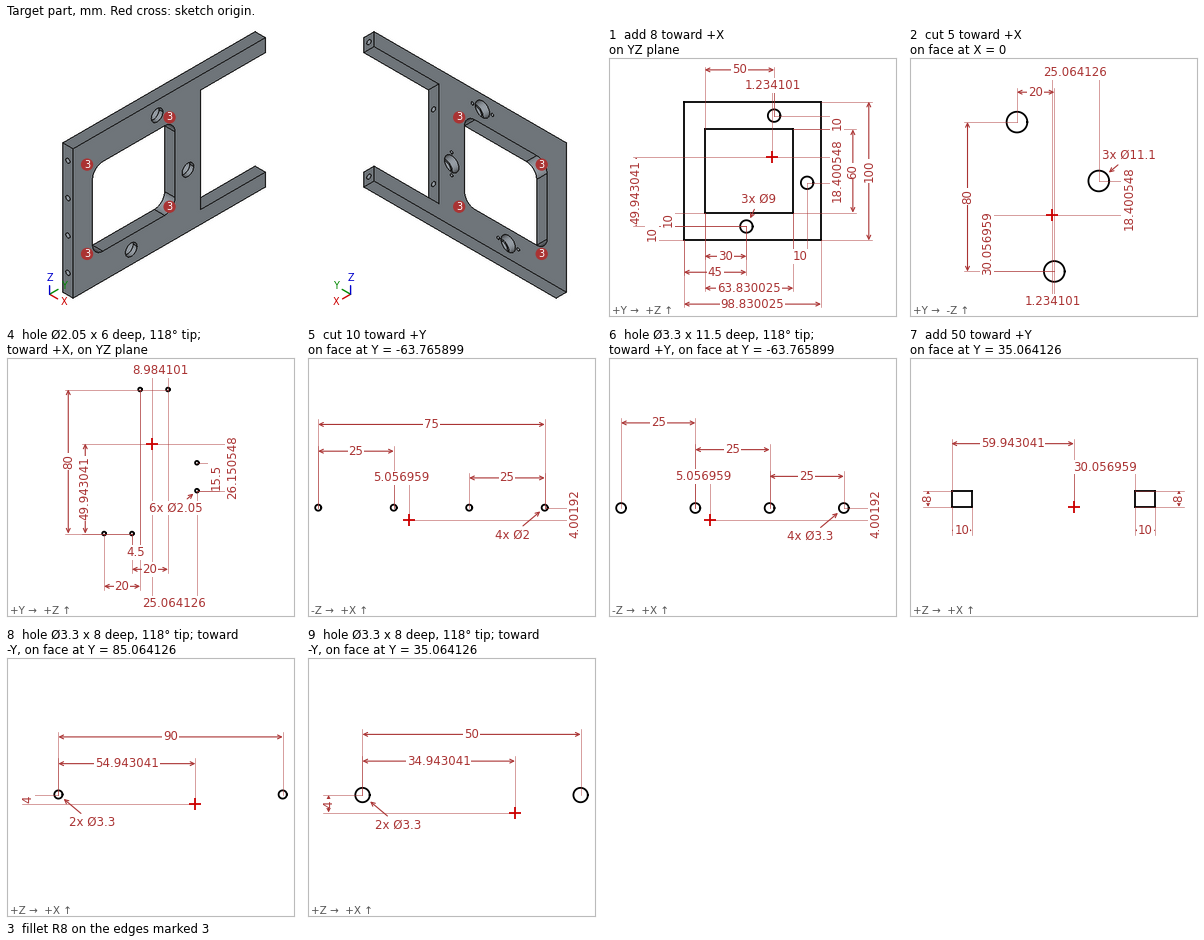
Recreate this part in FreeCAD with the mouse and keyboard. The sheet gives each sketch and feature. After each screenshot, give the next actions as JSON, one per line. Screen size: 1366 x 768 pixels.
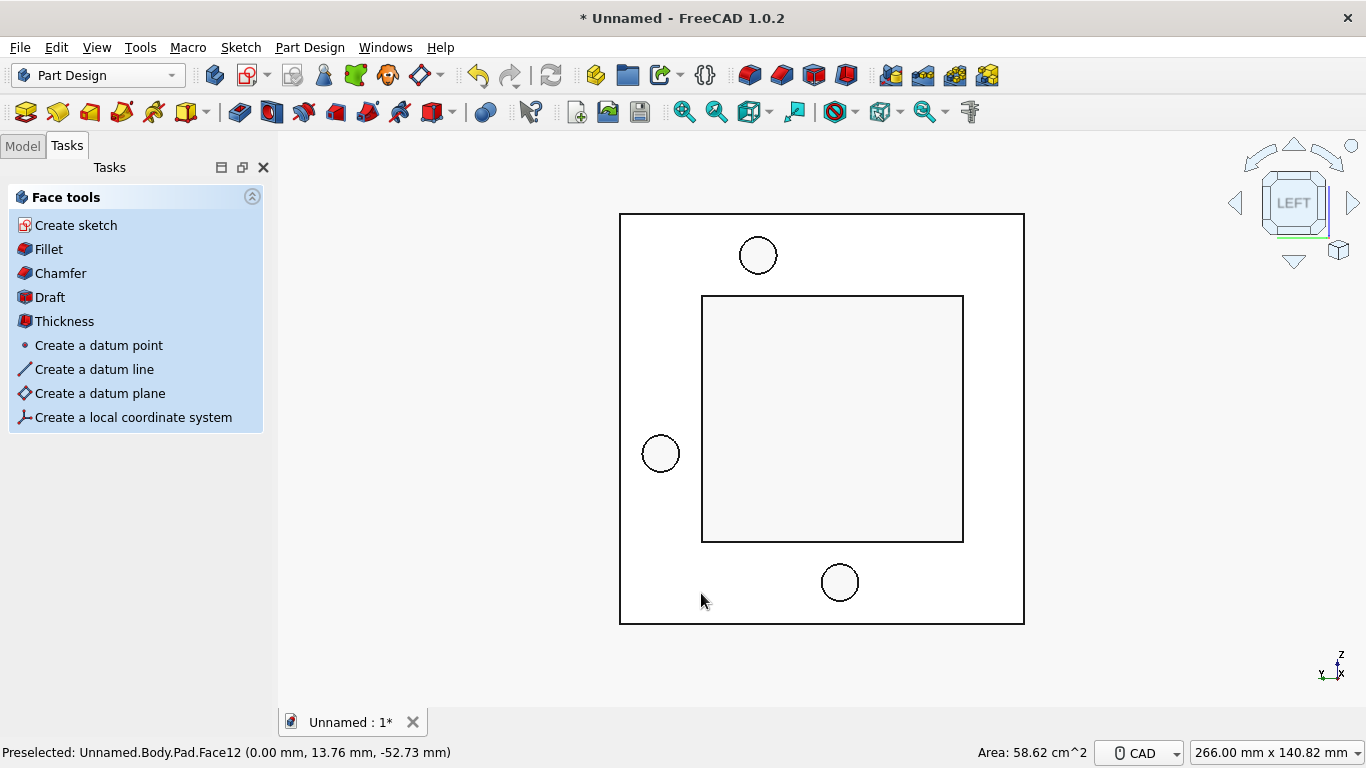
{"action": "left_click", "coordinate": [248, 76]}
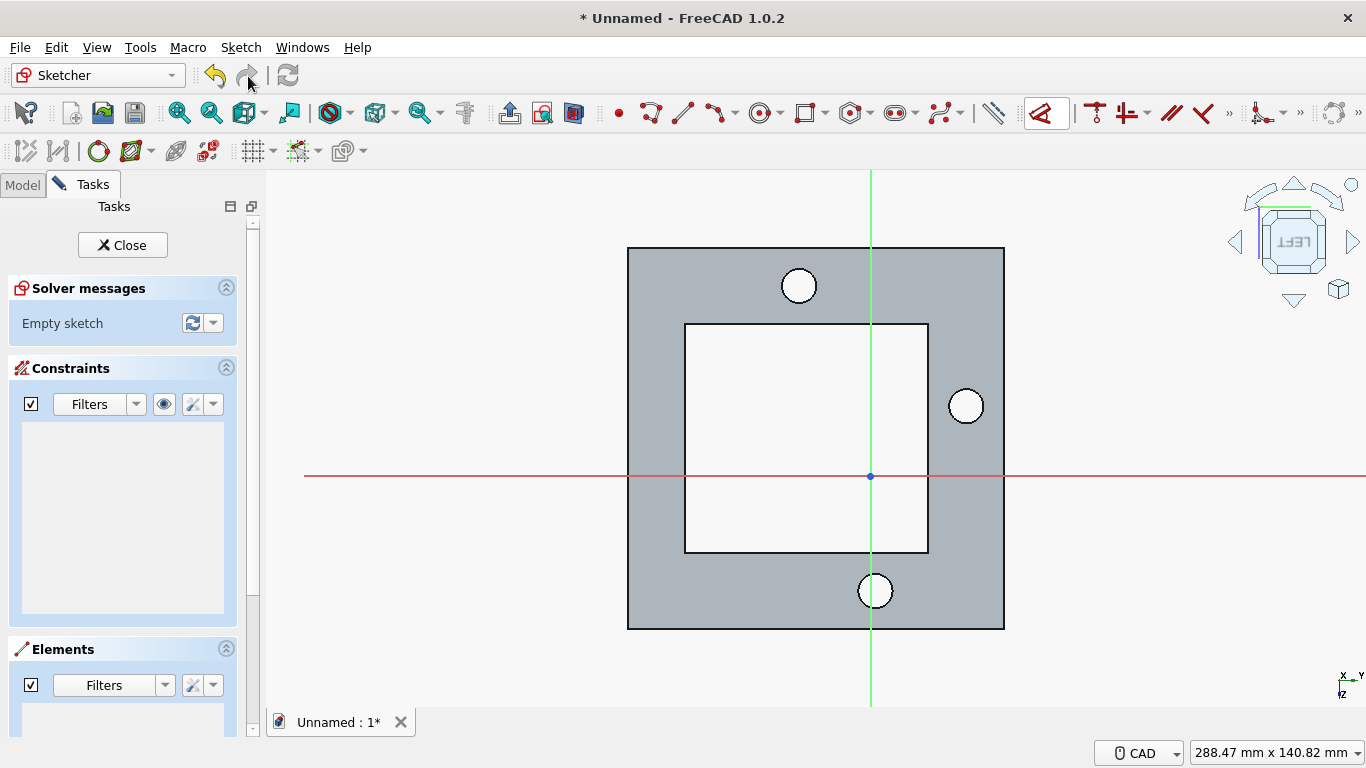
{"action": "key", "text": "g c"}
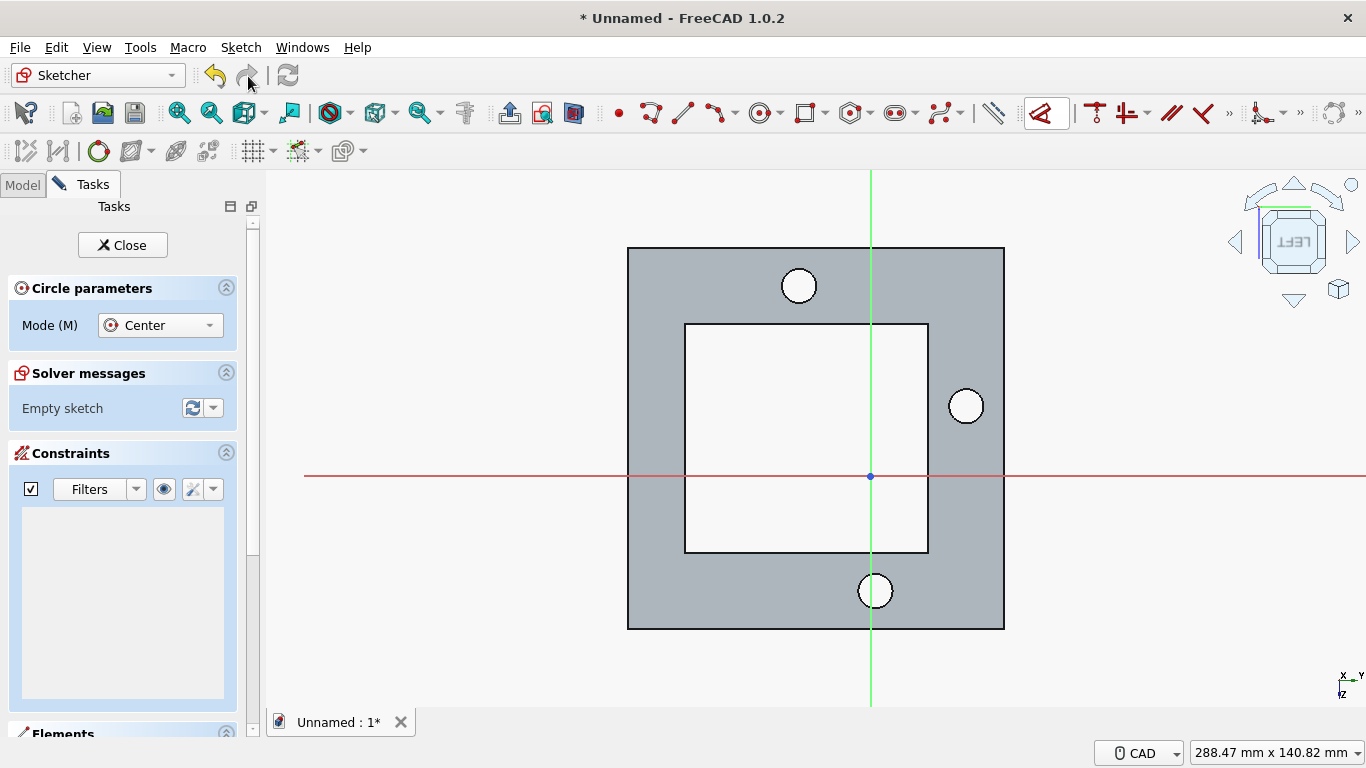
{"action": "left_click", "coordinate": [966, 406]}
{"action": "mouse_move", "coordinate": [981, 391]}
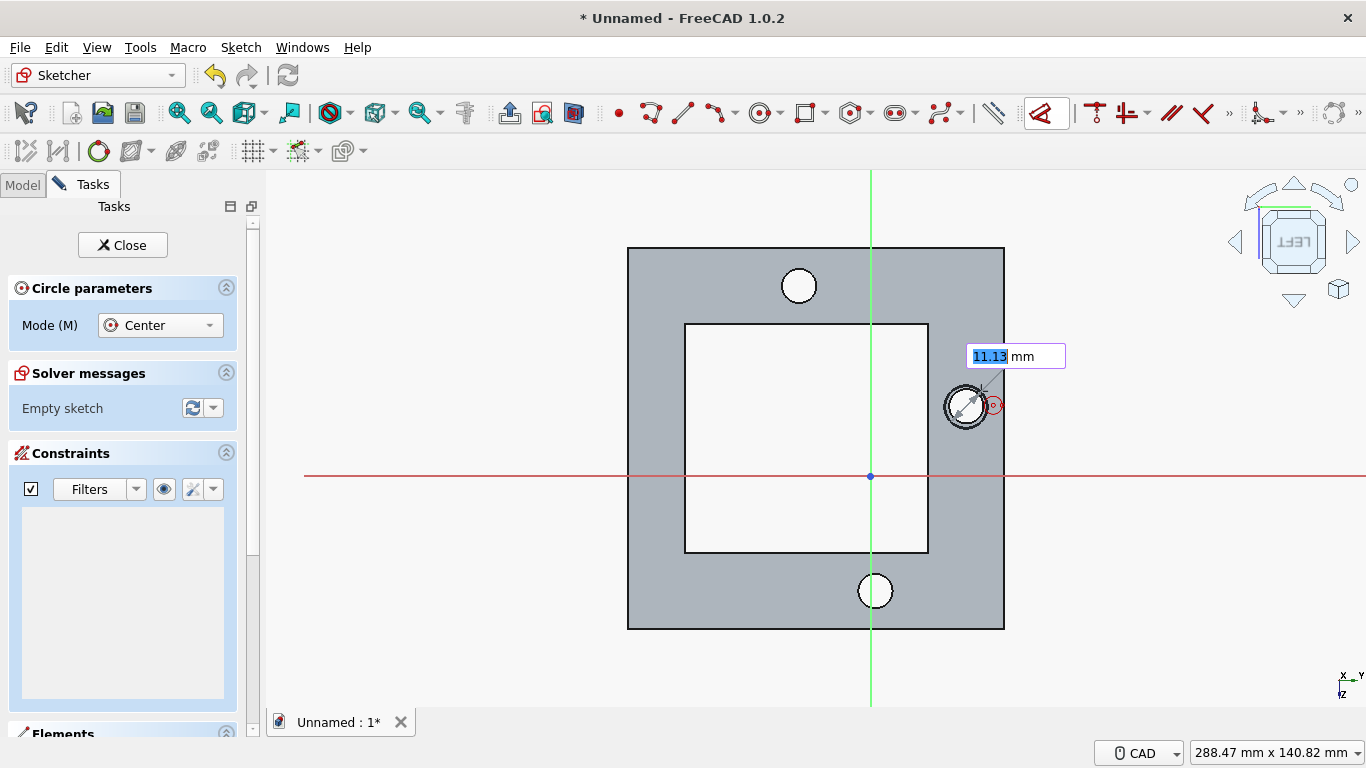
{"action": "type", "text": "11.1"}
{"action": "key", "text": "Return"}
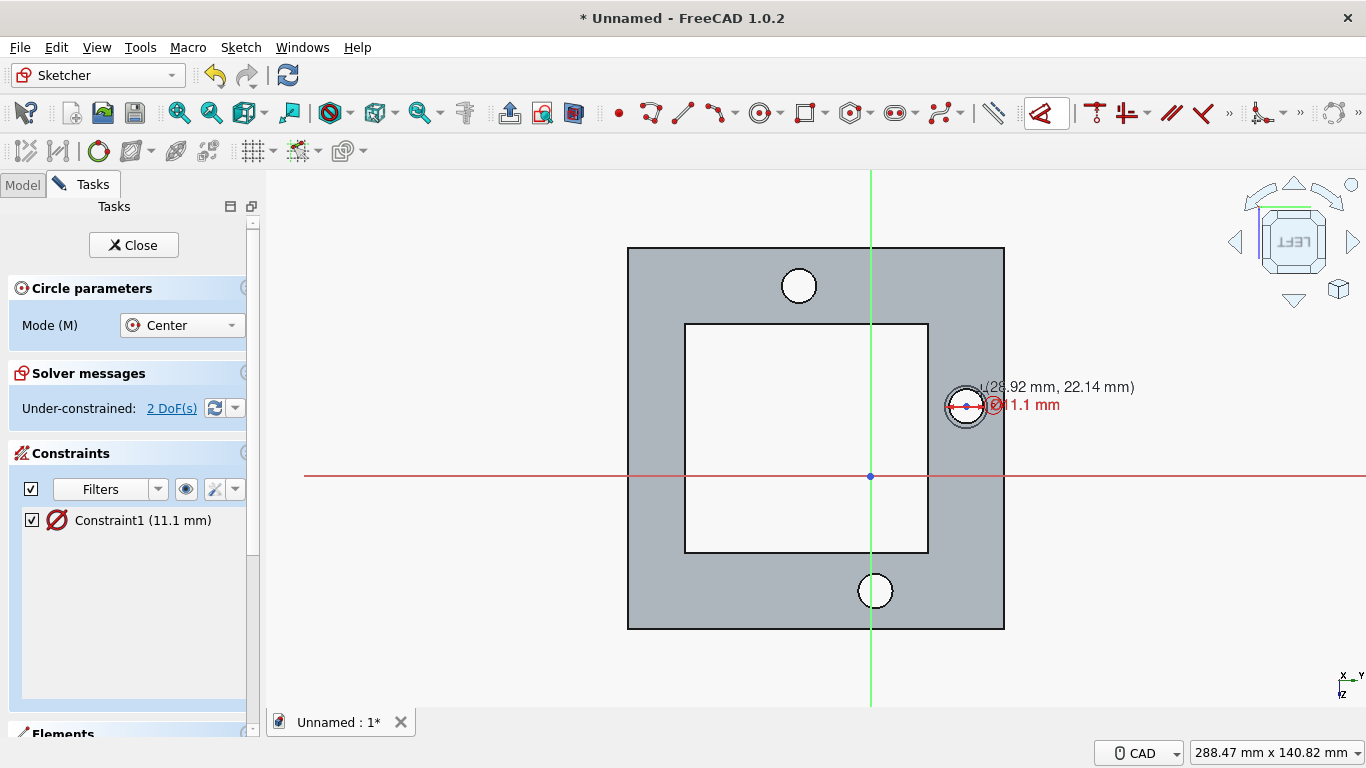
{"action": "scroll", "coordinate": [875, 591], "scroll_direction": "up", "scroll_amount": 7}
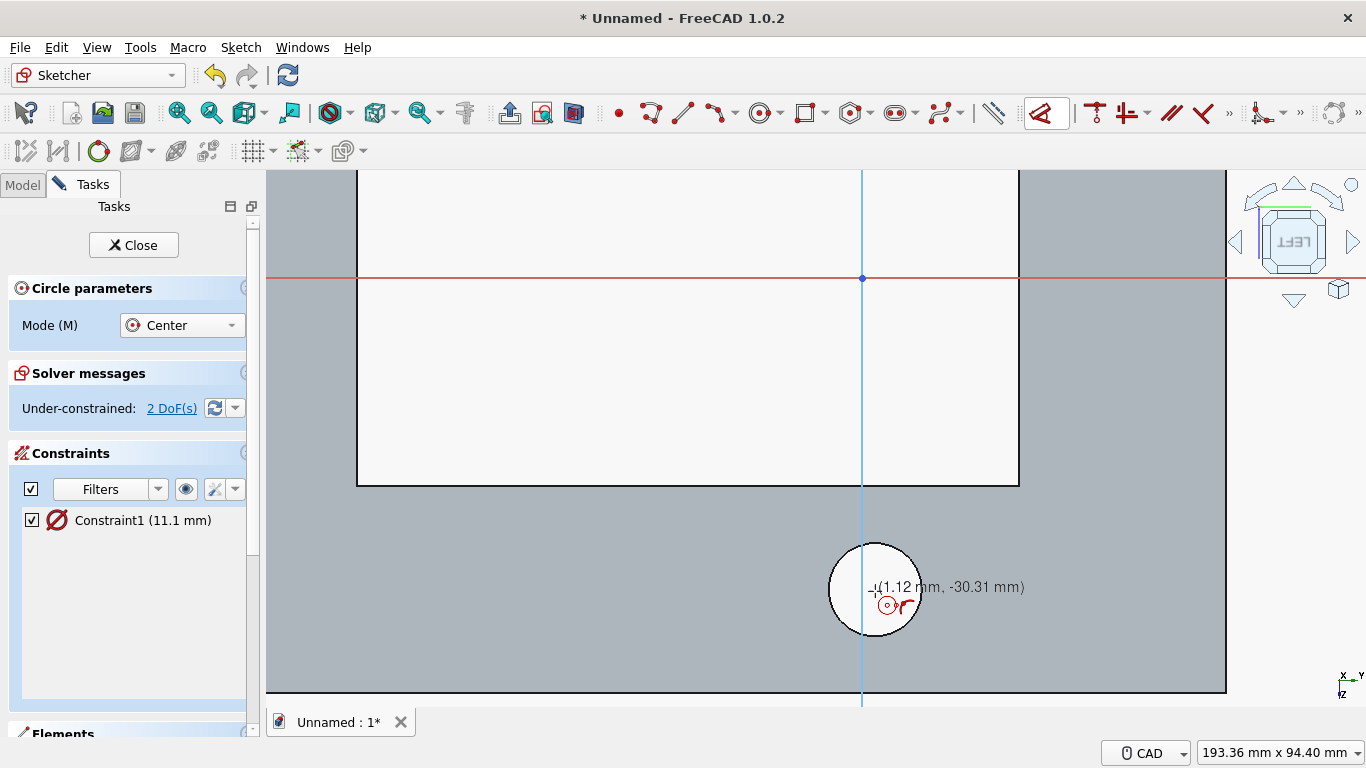
{"action": "left_click", "coordinate": [875, 589]}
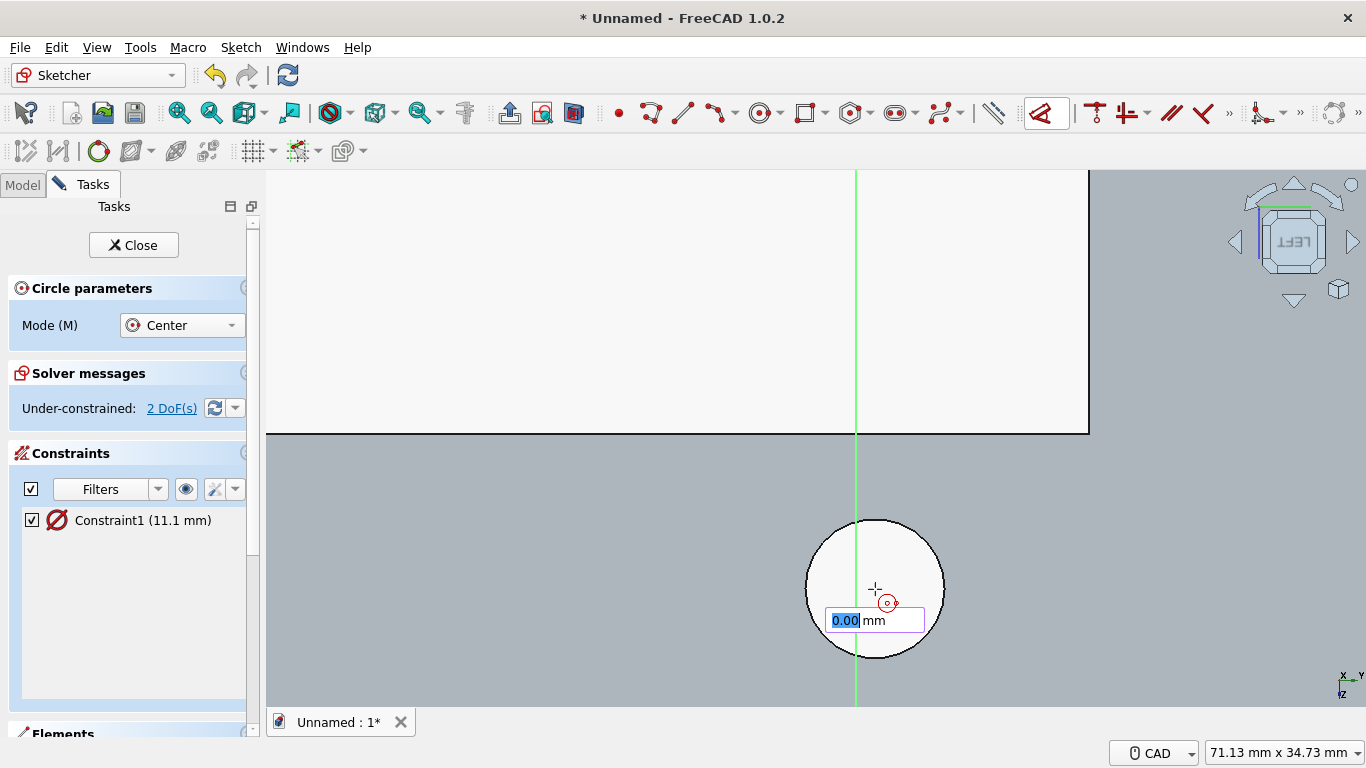
{"action": "scroll", "coordinate": [696, 592], "scroll_direction": "down", "scroll_amount": 7}
{"action": "mouse_move", "coordinate": [755, 577]}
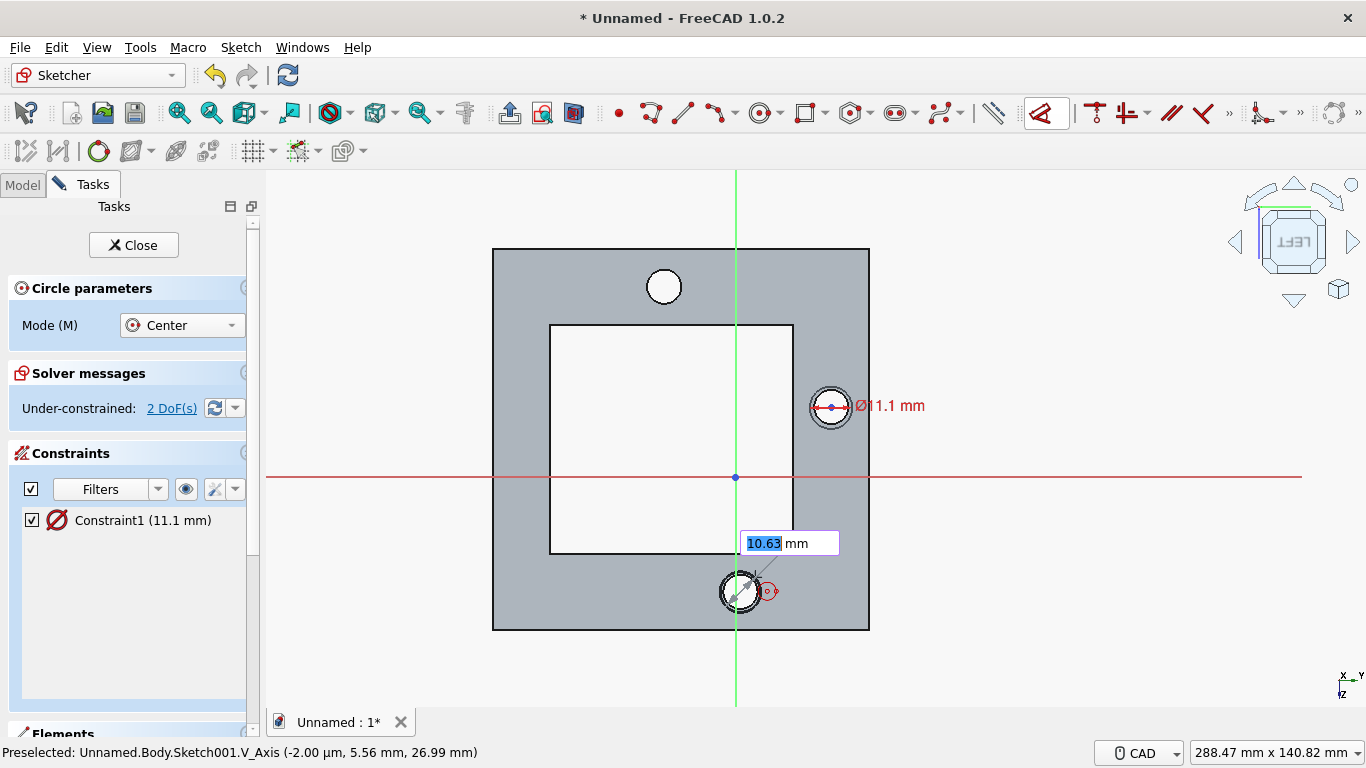
{"action": "type", "text": "11.1"}
{"action": "key", "text": "Return"}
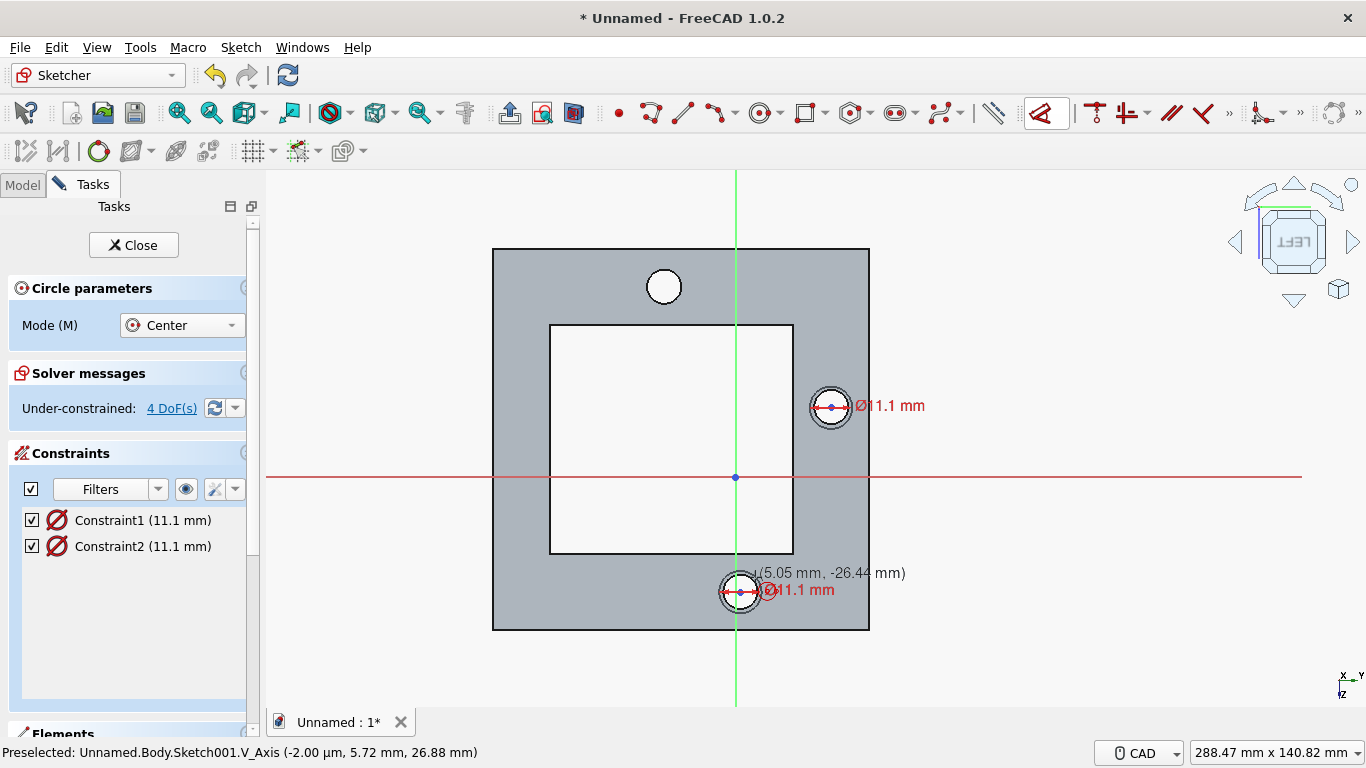
{"action": "left_click", "coordinate": [664, 287]}
{"action": "mouse_move", "coordinate": [679, 272]}